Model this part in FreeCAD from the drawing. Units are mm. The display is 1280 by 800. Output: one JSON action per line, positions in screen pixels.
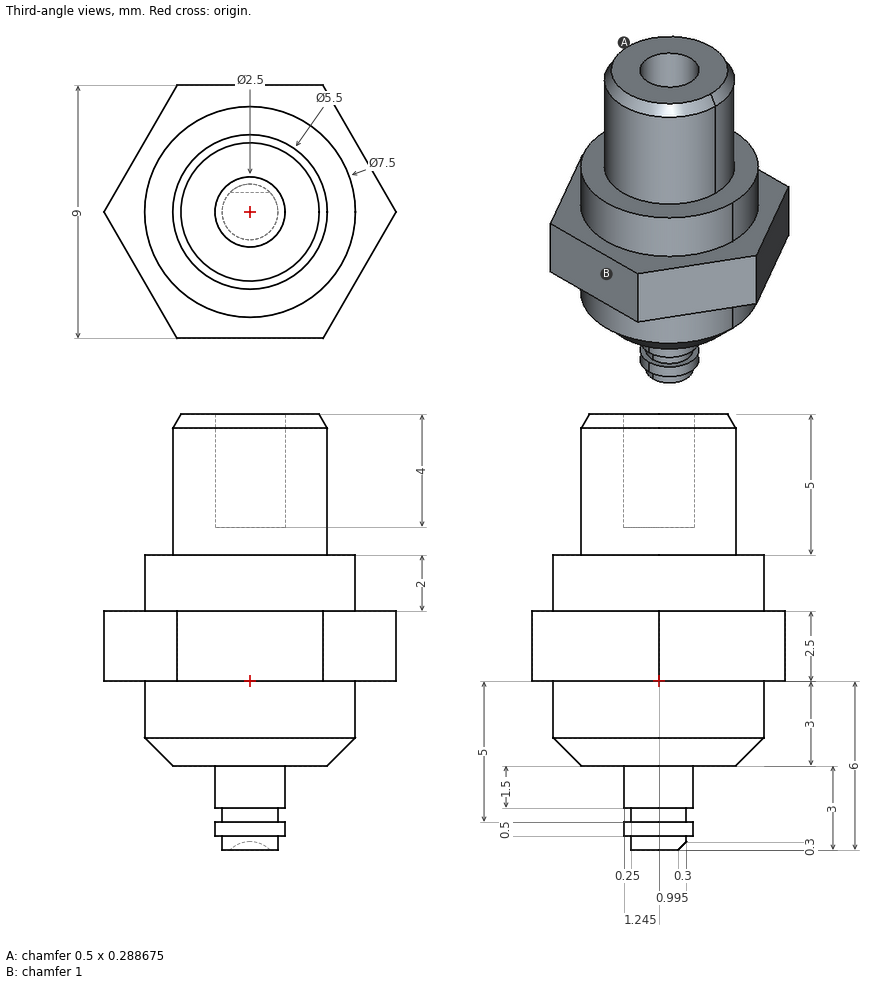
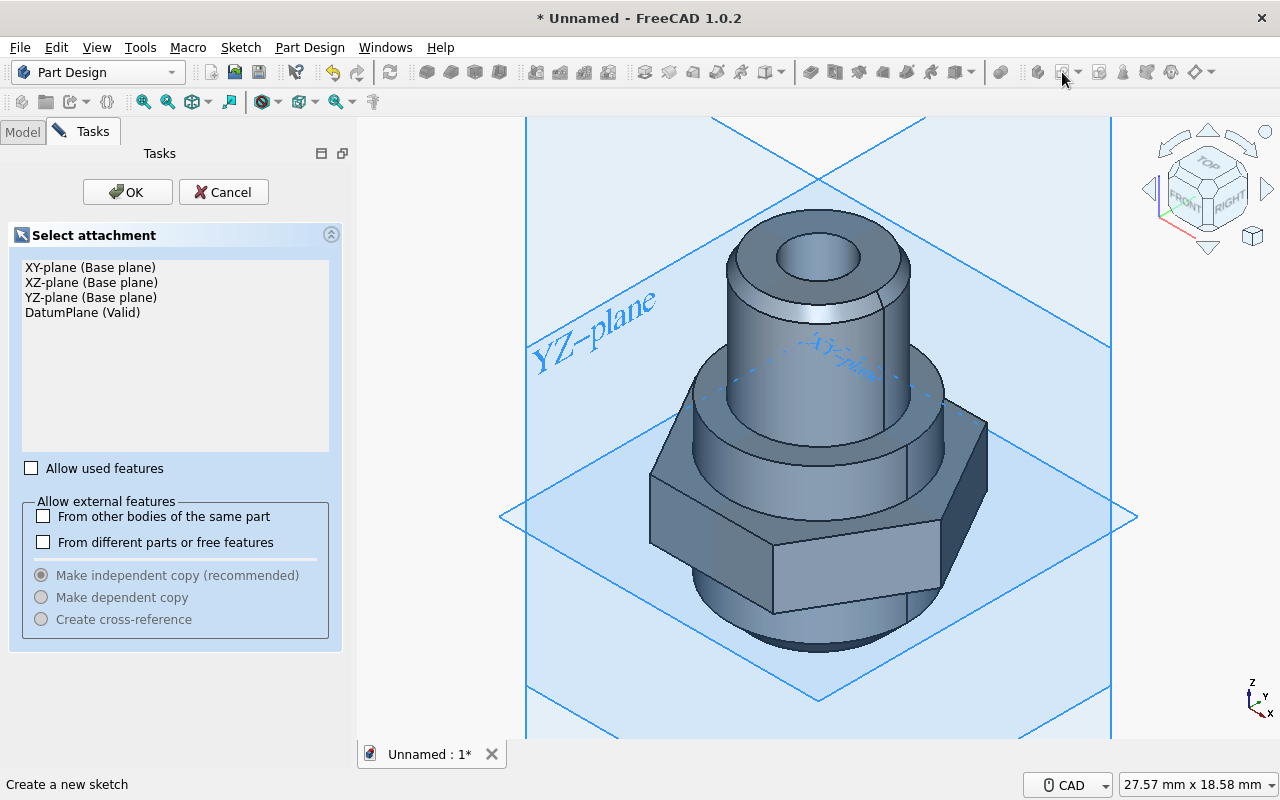
{"action": "left_click", "coordinate": [82, 298]}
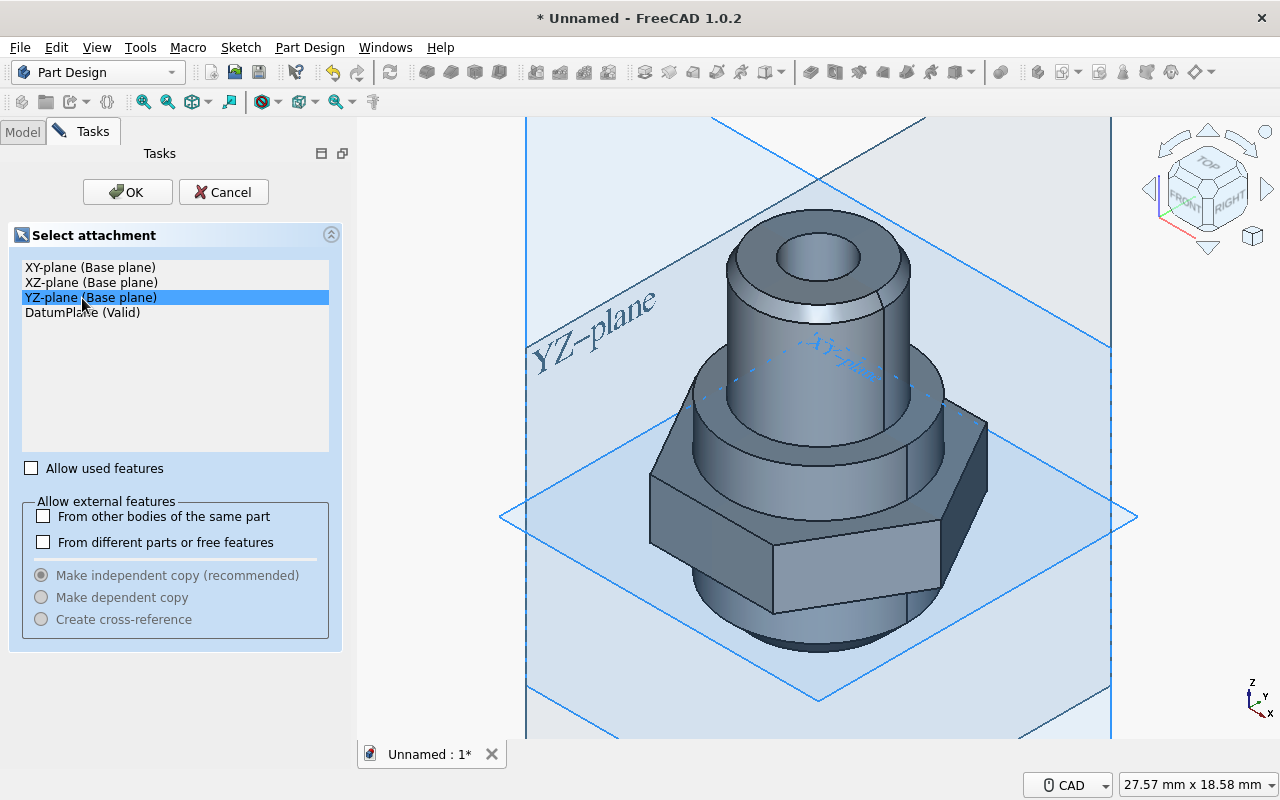
{"action": "left_click", "coordinate": [128, 192]}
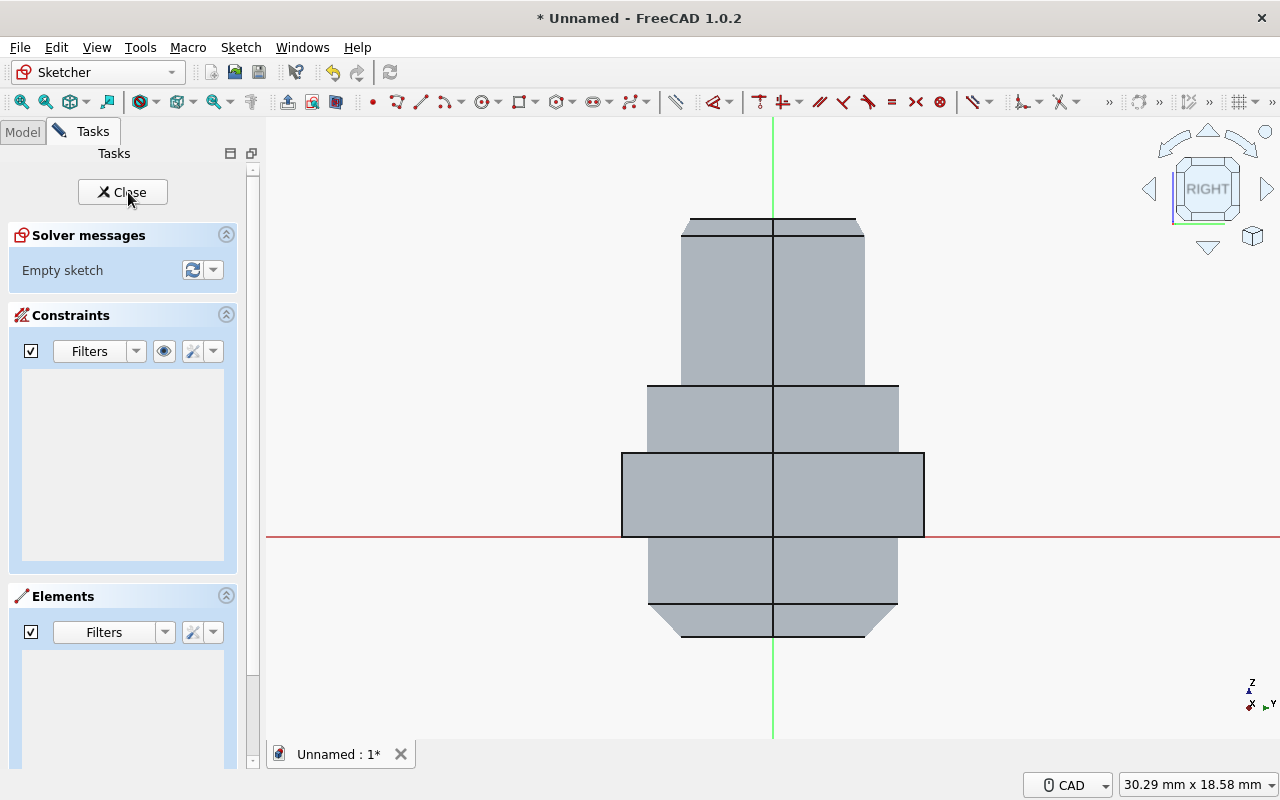
{"action": "left_click", "coordinate": [336, 102]}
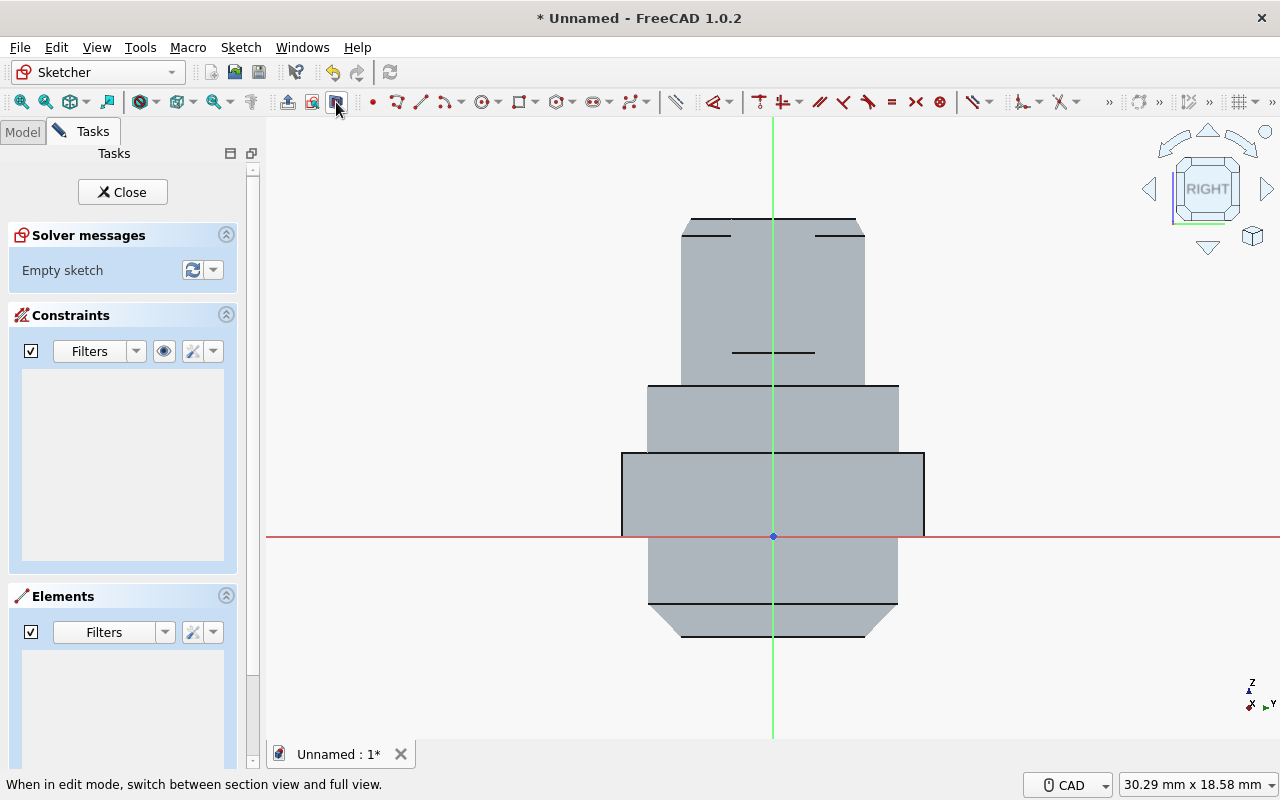
{"action": "scroll", "coordinate": [704, 428], "scroll_direction": "down", "scroll_amount": 5}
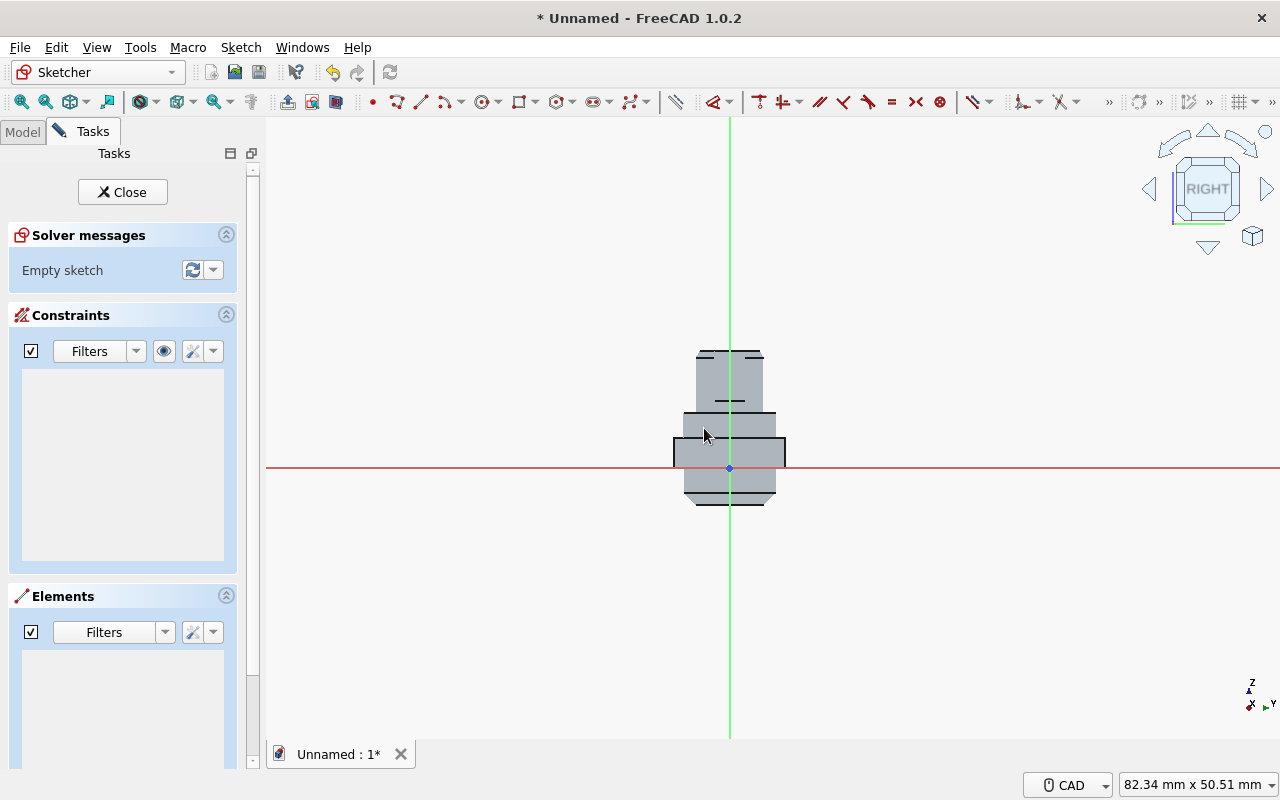
{"action": "scroll", "coordinate": [726, 525], "scroll_direction": "up", "scroll_amount": 8}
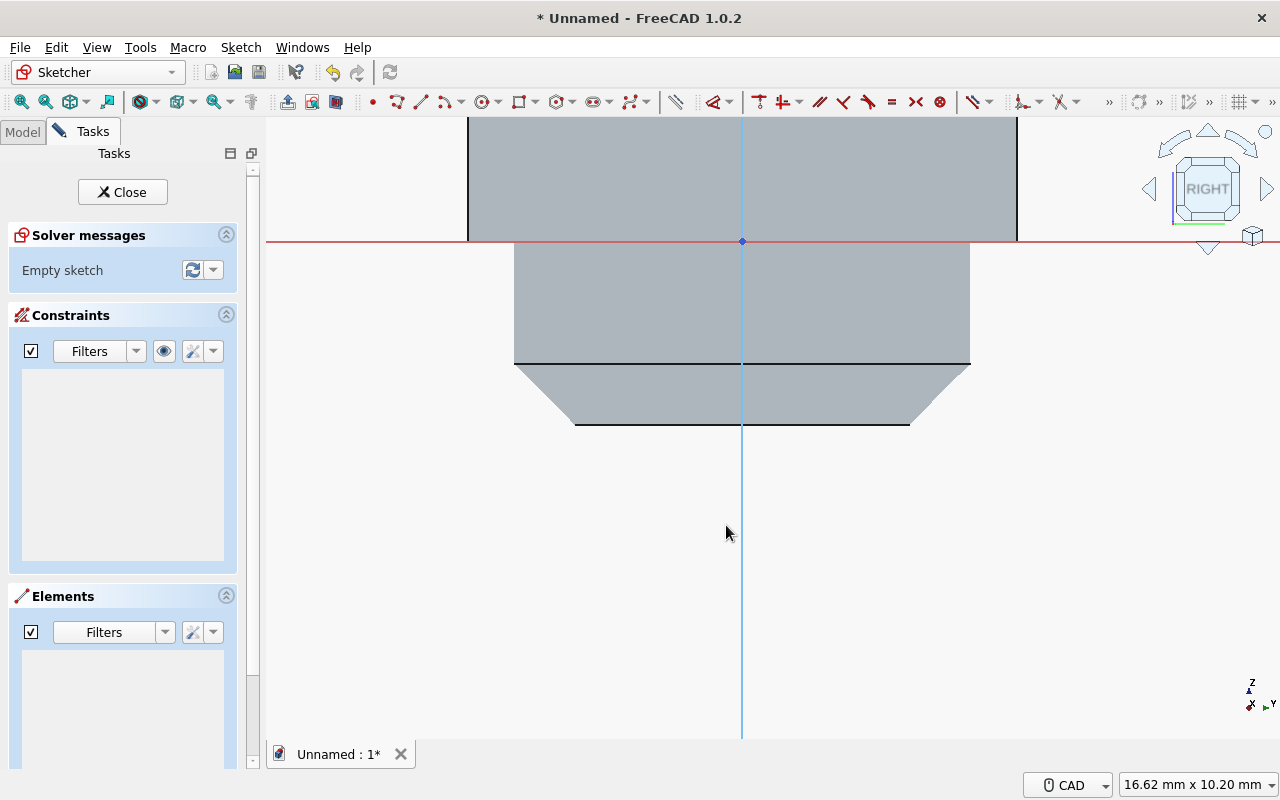
{"action": "key", "text": "g m"}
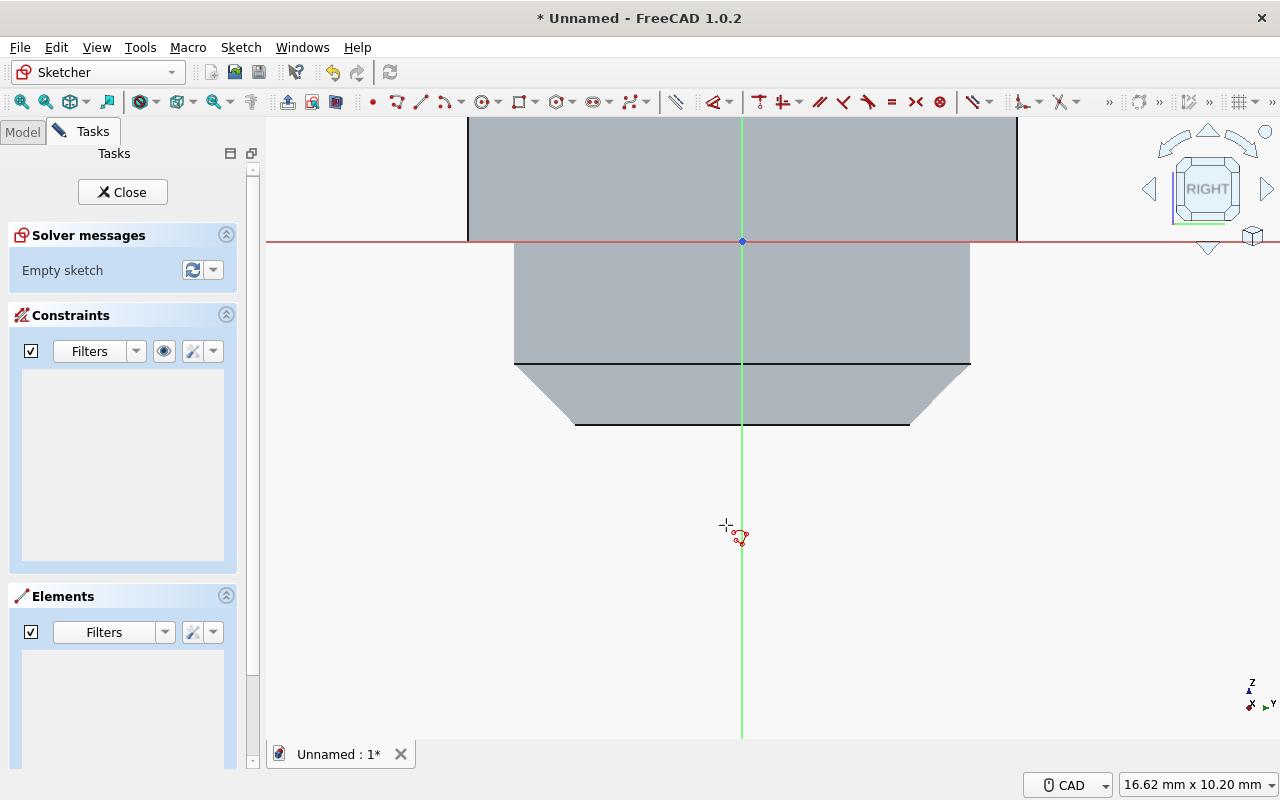
{"action": "left_click", "coordinate": [742, 425]}
{"action": "left_click", "coordinate": [666, 425]}
{"action": "left_click", "coordinate": [666, 516]}
{"action": "left_click", "coordinate": [682, 516]}
{"action": "left_click", "coordinate": [682, 547]}
{"action": "left_click", "coordinate": [666, 547]}
{"action": "left_click", "coordinate": [666, 577]}
{"action": "left_click", "coordinate": [682, 577]}
{"action": "left_click", "coordinate": [682, 608]}
{"action": "left_click", "coordinate": [733, 608]}
{"action": "left_click", "coordinate": [742, 426]}
{"action": "key", "text": "Escape"}
{"action": "key", "text": "Escape"}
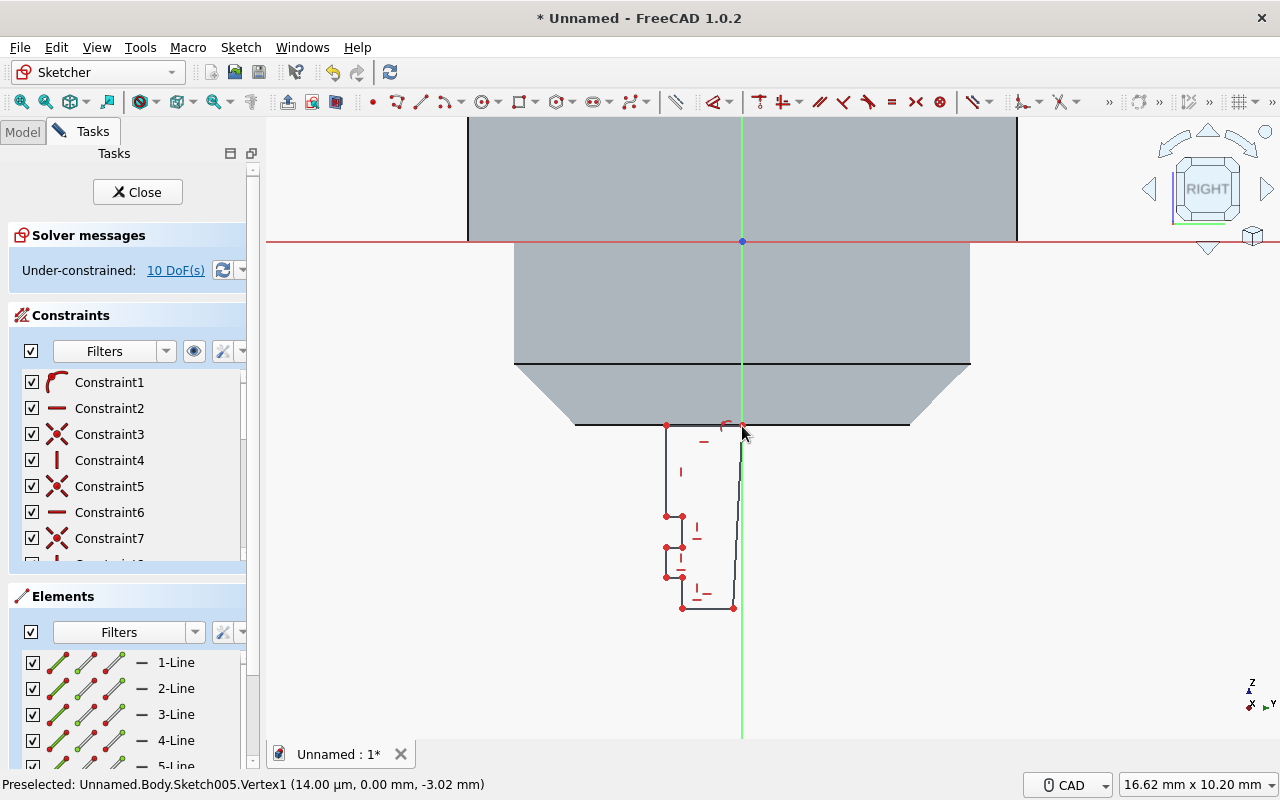
{"action": "left_click", "coordinate": [740, 481]}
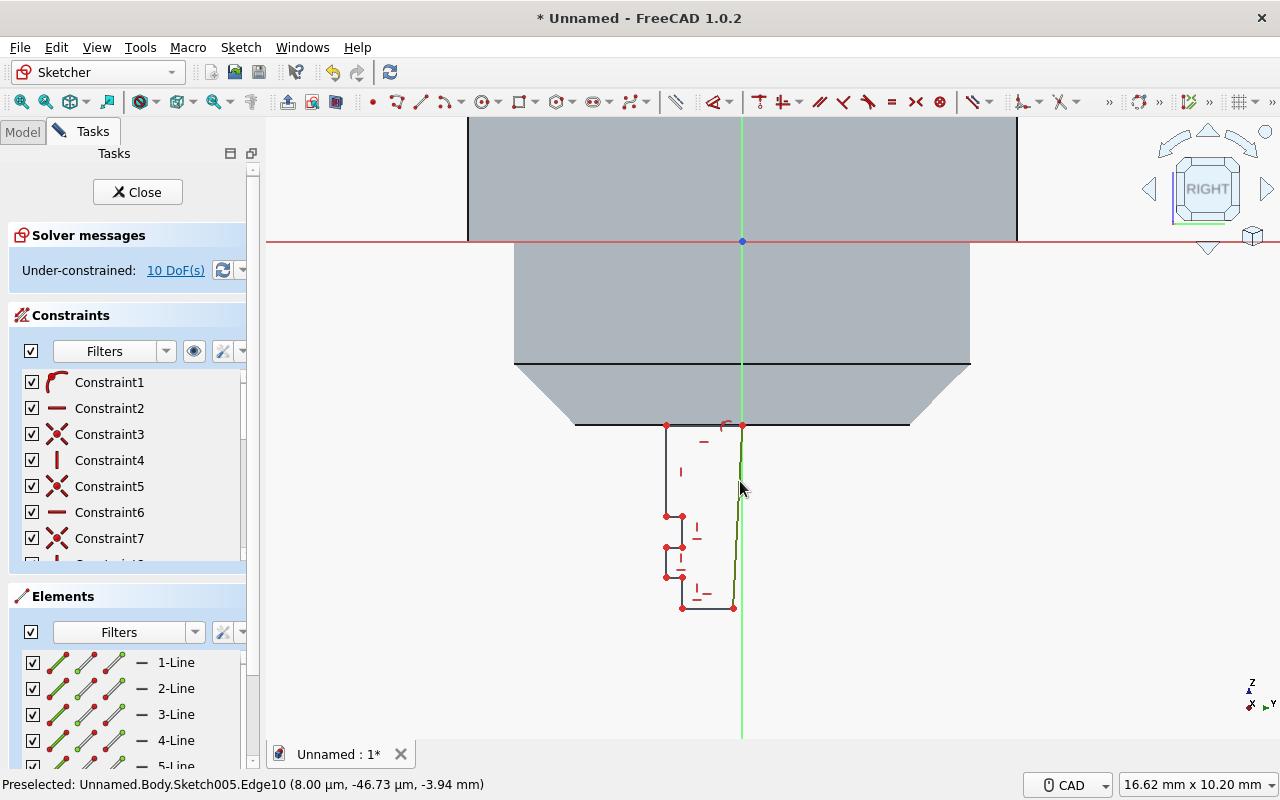
{"action": "key", "text": "v"}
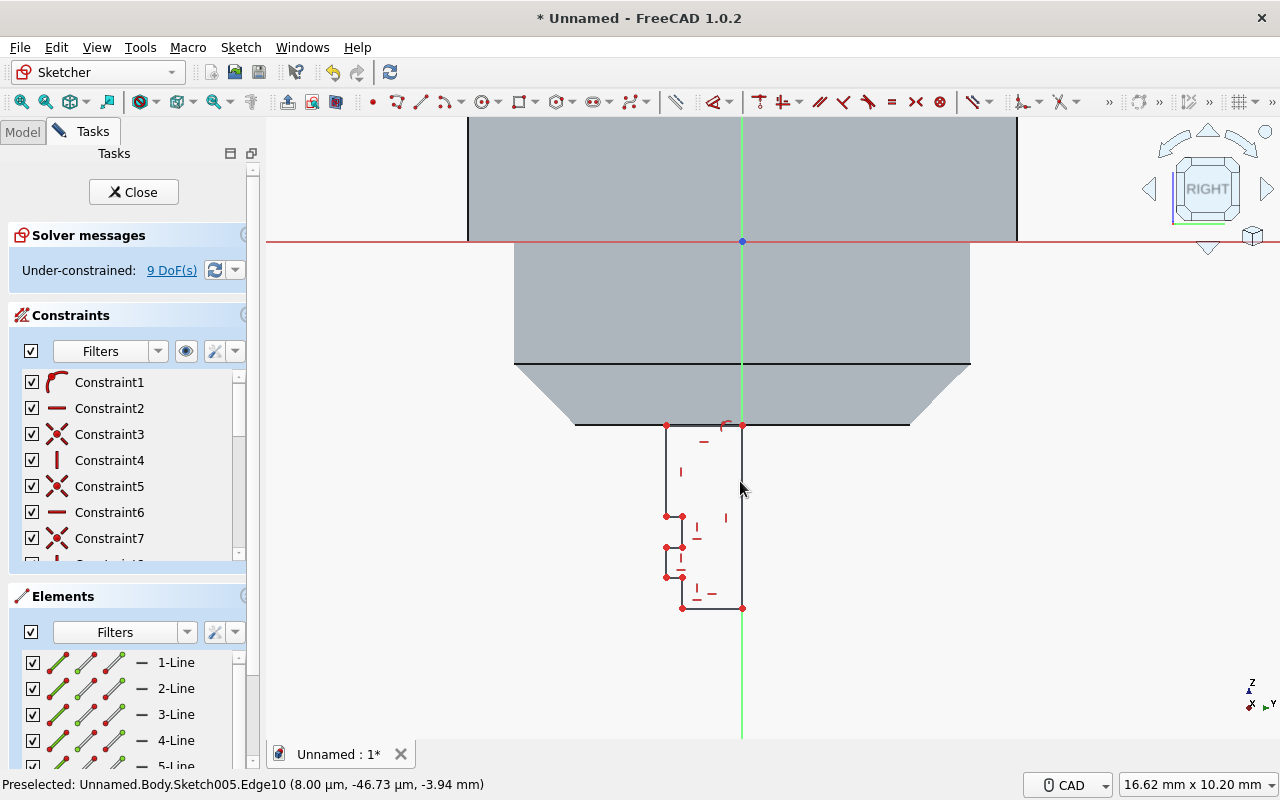
{"action": "left_click", "coordinate": [742, 554]}